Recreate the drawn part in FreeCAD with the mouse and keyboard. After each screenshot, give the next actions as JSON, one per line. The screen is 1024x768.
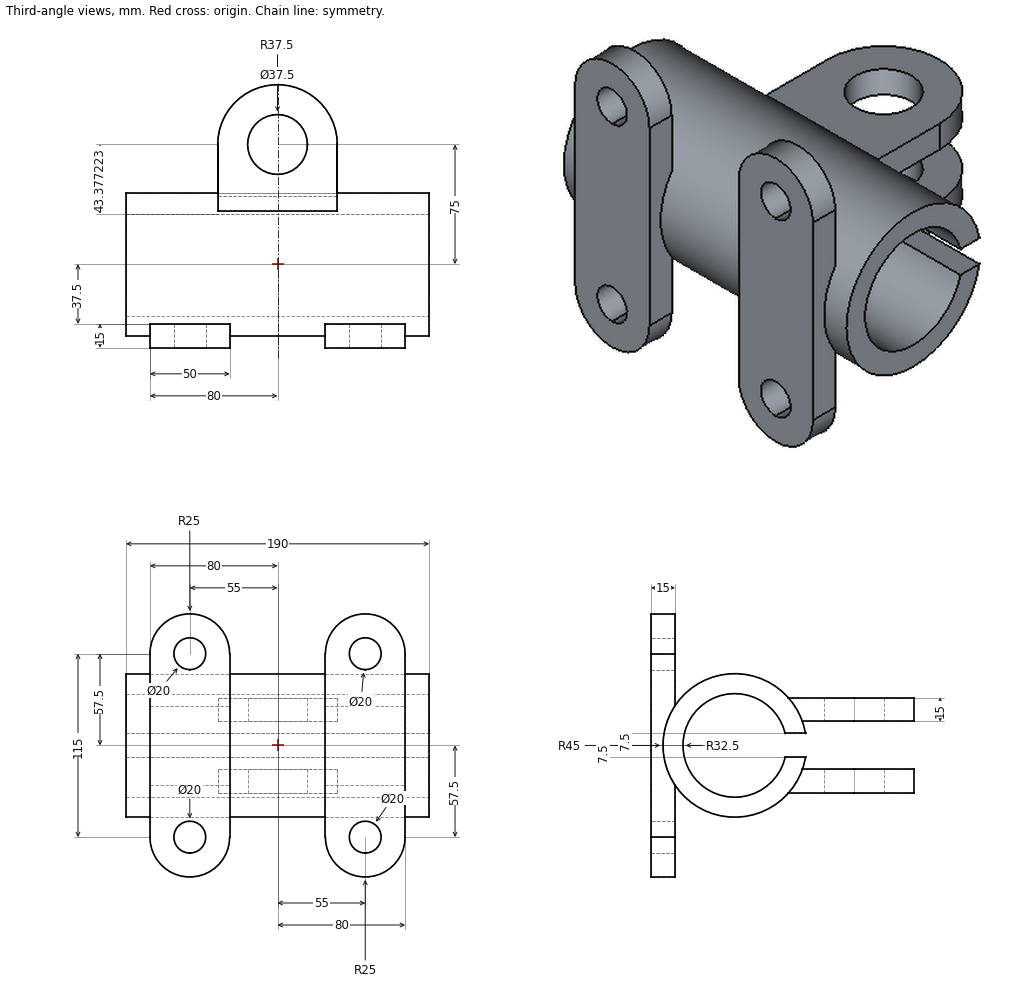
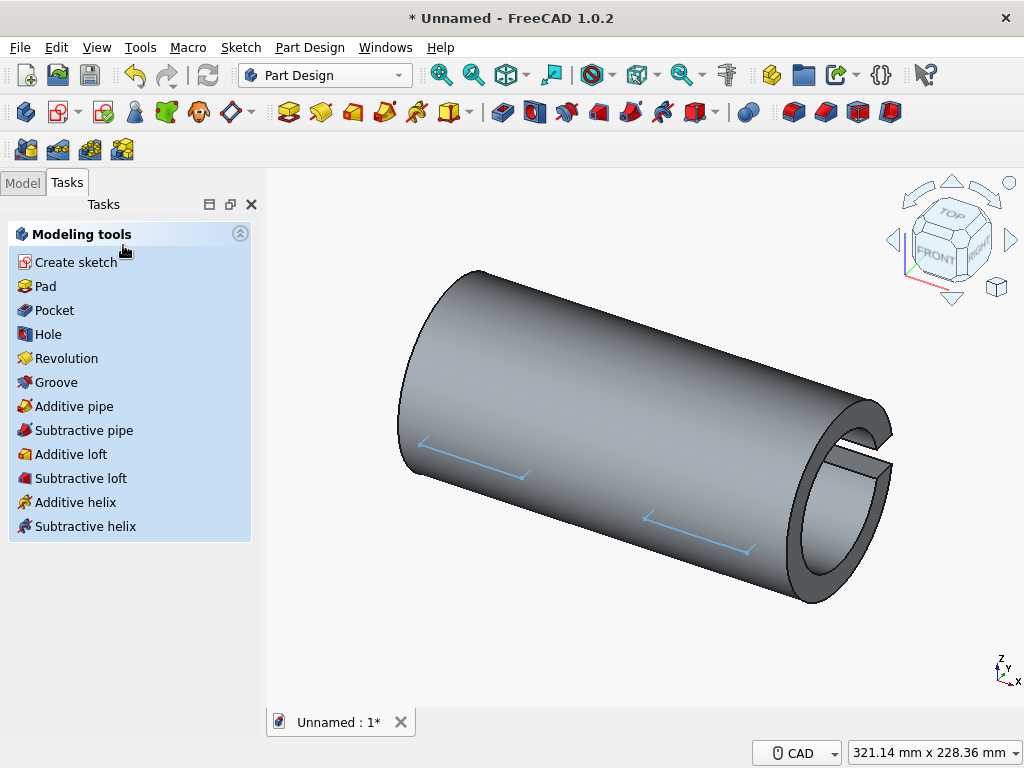
{"action": "left_click", "coordinate": [290, 112]}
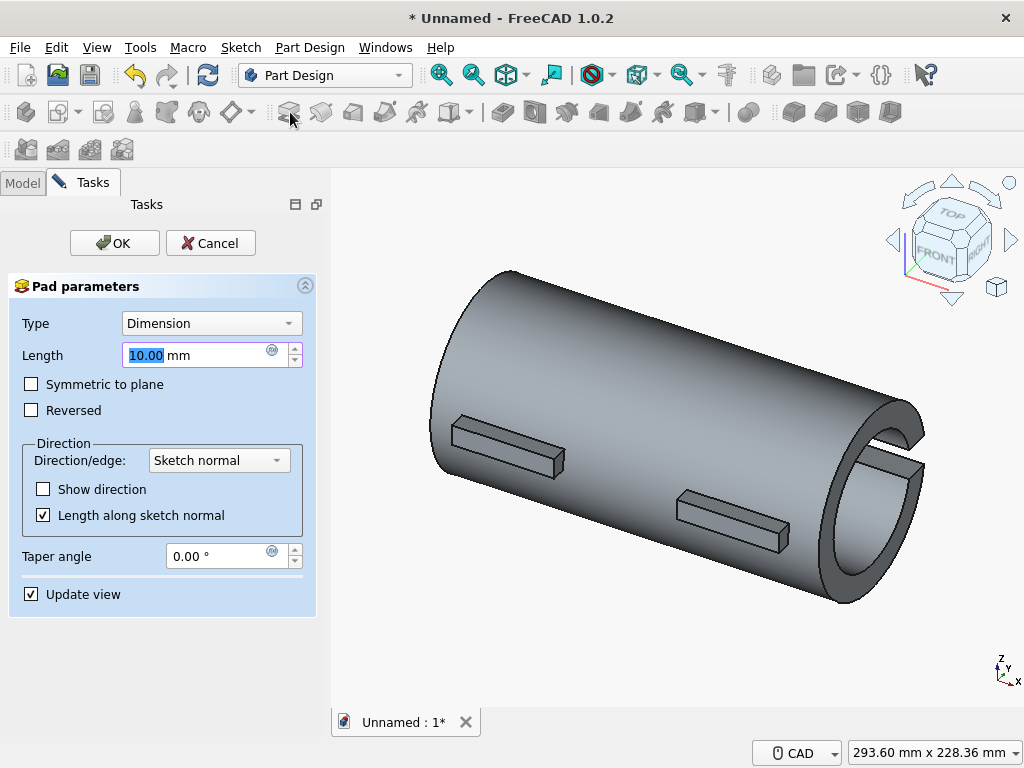
{"action": "type", "text": "115"}
{"action": "key", "text": "Tab"}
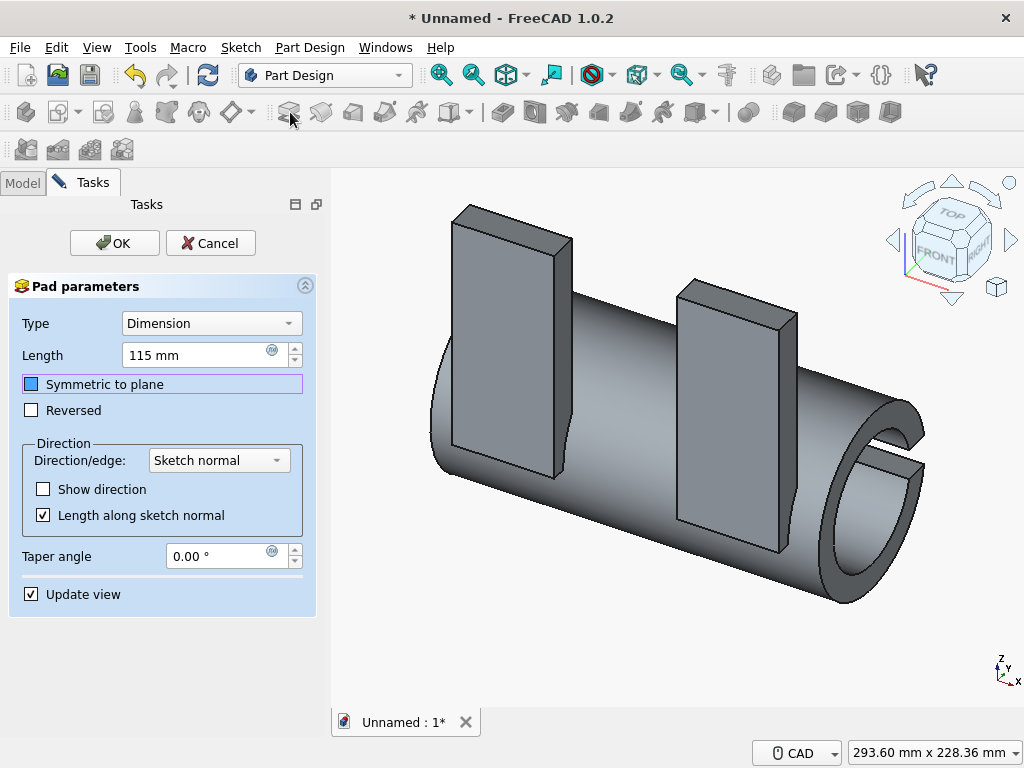
{"action": "left_click", "coordinate": [30, 384]}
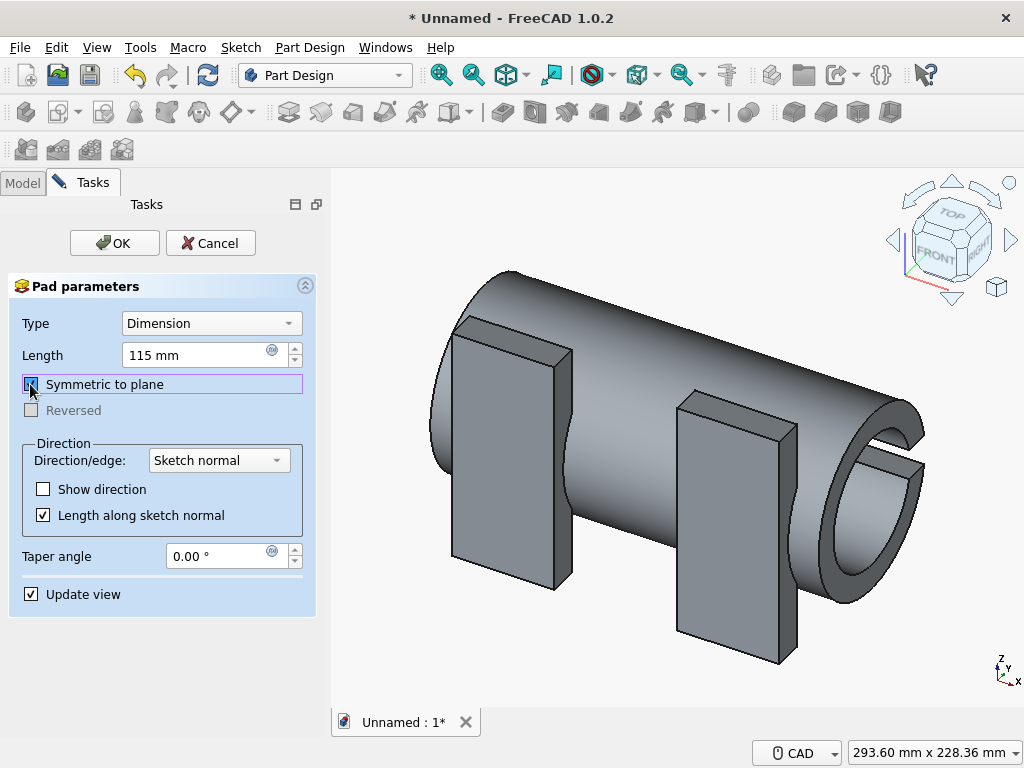
{"action": "left_click", "coordinate": [115, 243]}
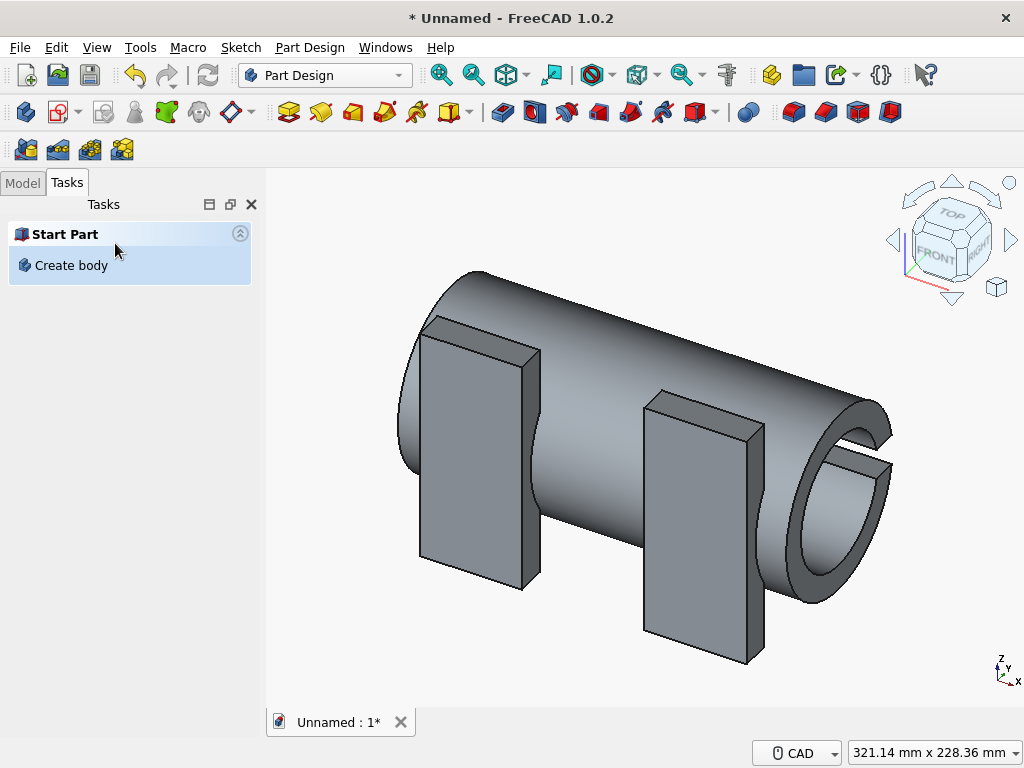
{"action": "left_click", "coordinate": [471, 429]}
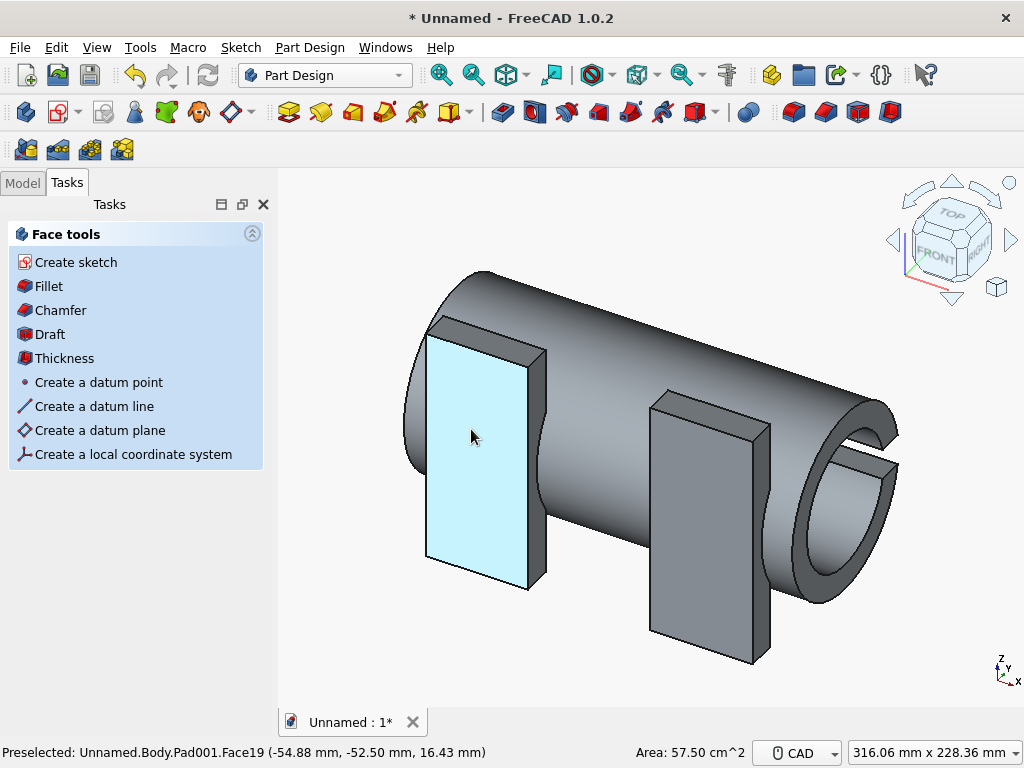
{"action": "left_click", "coordinate": [58, 112]}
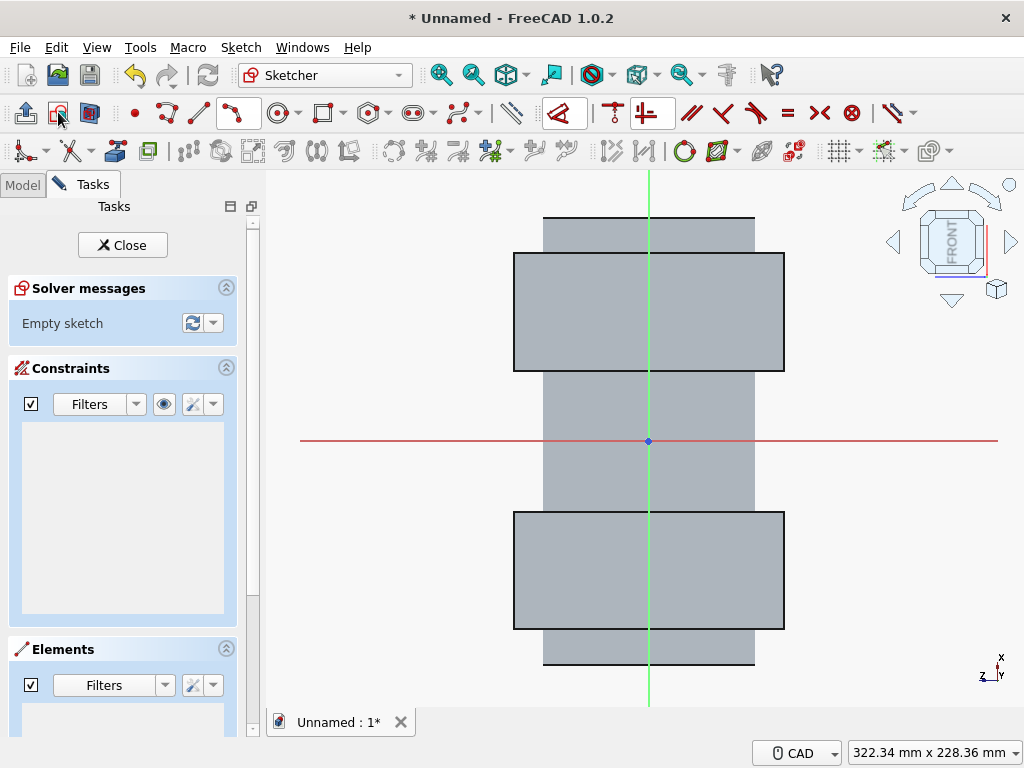
{"action": "scroll", "coordinate": [522, 653], "scroll_direction": "up", "scroll_amount": 3}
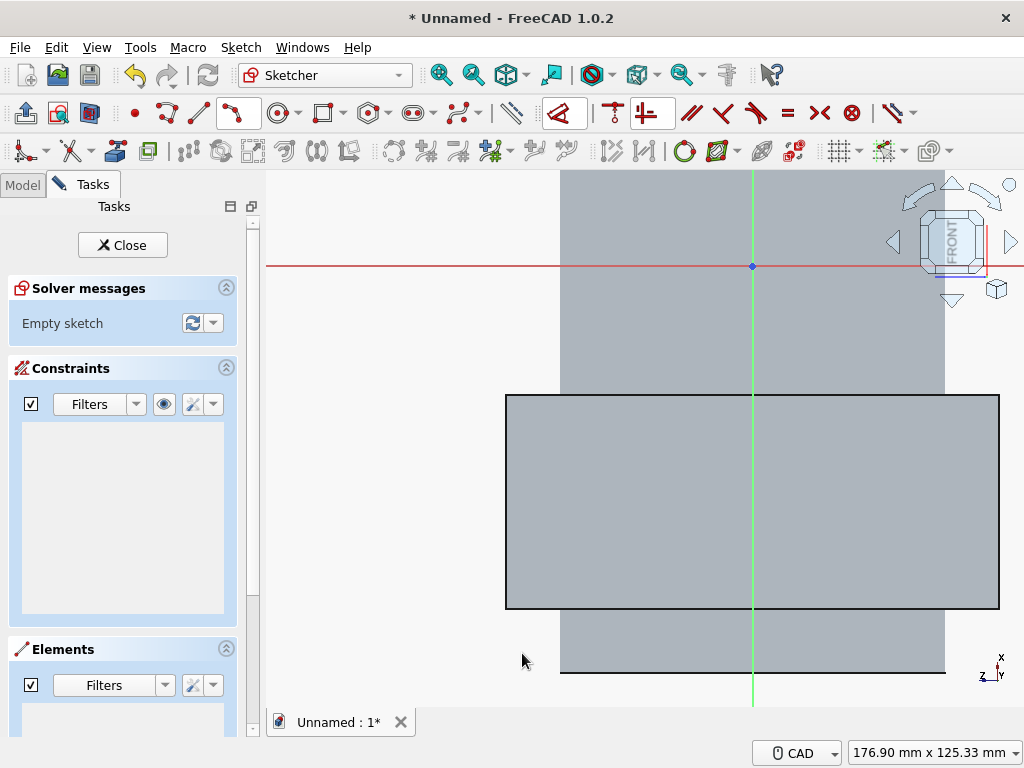
{"action": "left_click", "coordinate": [200, 114]}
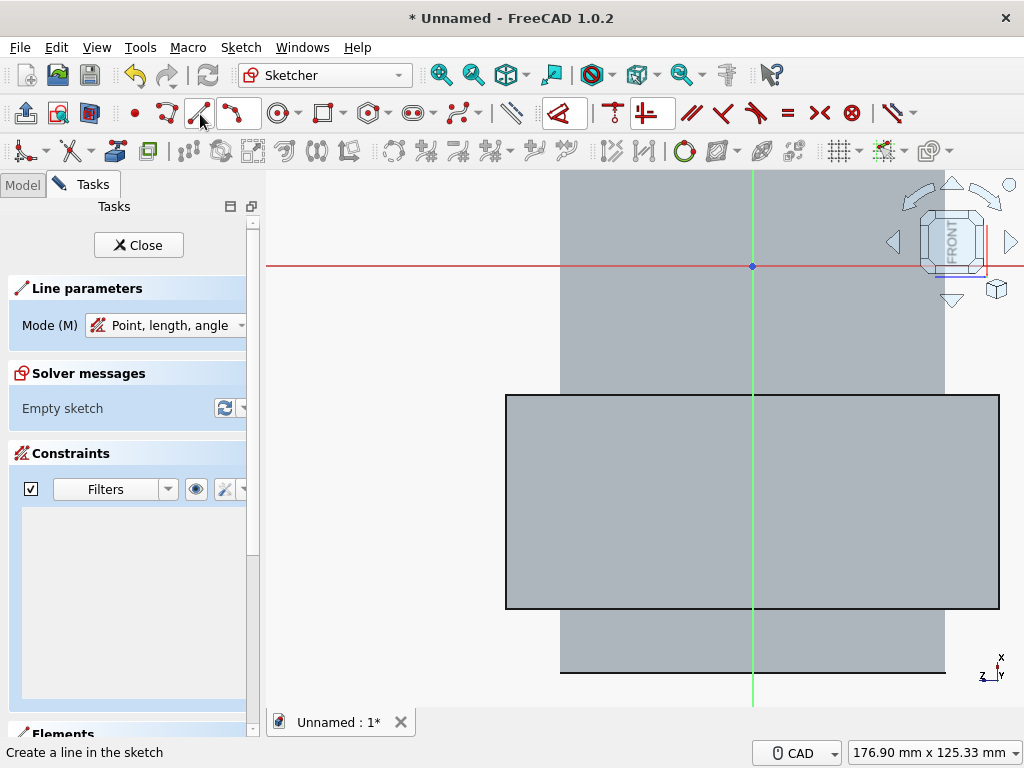
{"action": "left_click", "coordinate": [506, 609]}
{"action": "left_click", "coordinate": [506, 395]}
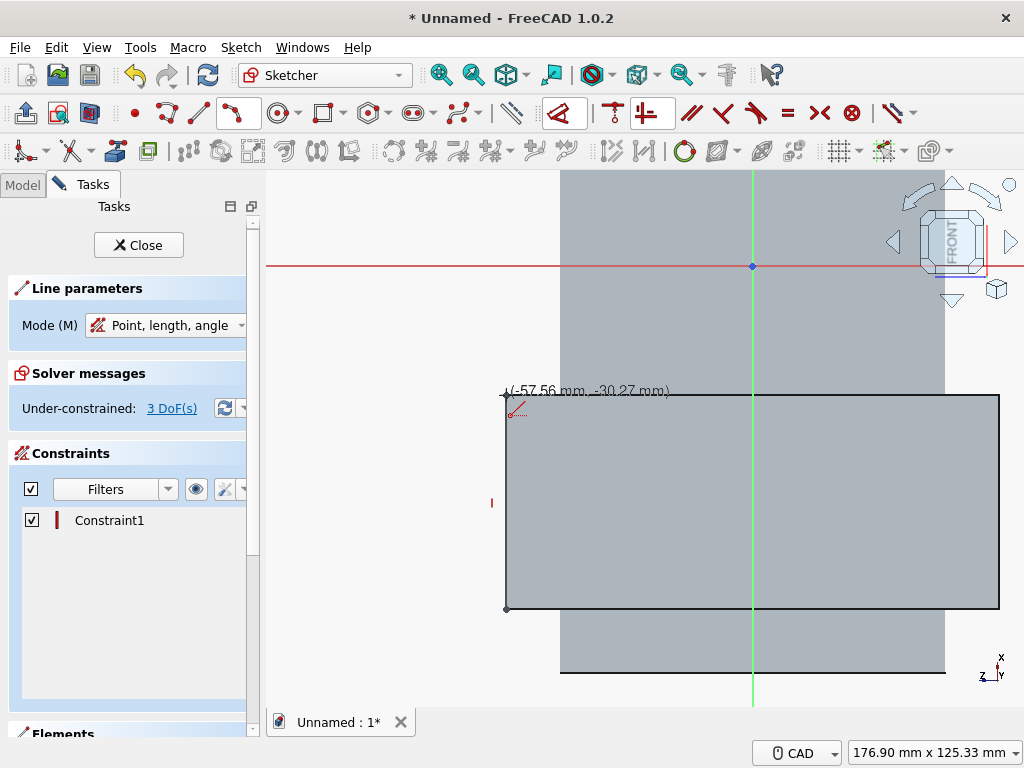
{"action": "left_click", "coordinate": [232, 114]}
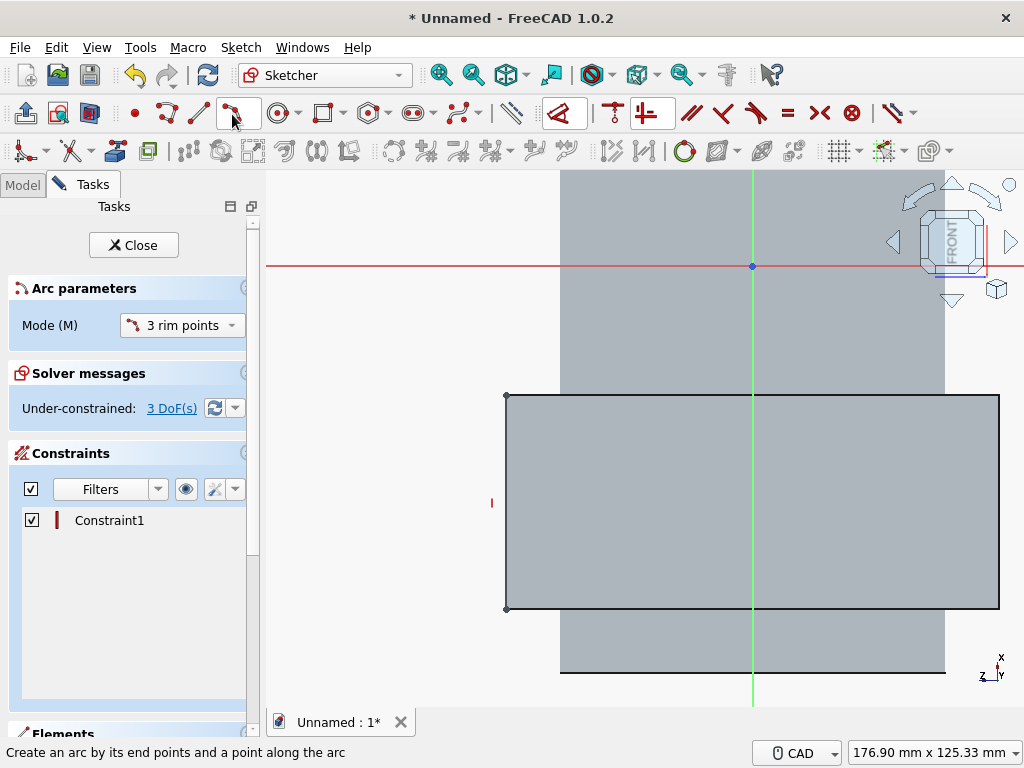
{"action": "left_click", "coordinate": [506, 396]}
{"action": "left_click", "coordinate": [506, 610]}
{"action": "left_click", "coordinate": [399, 502]}
{"action": "key", "text": "Escape"}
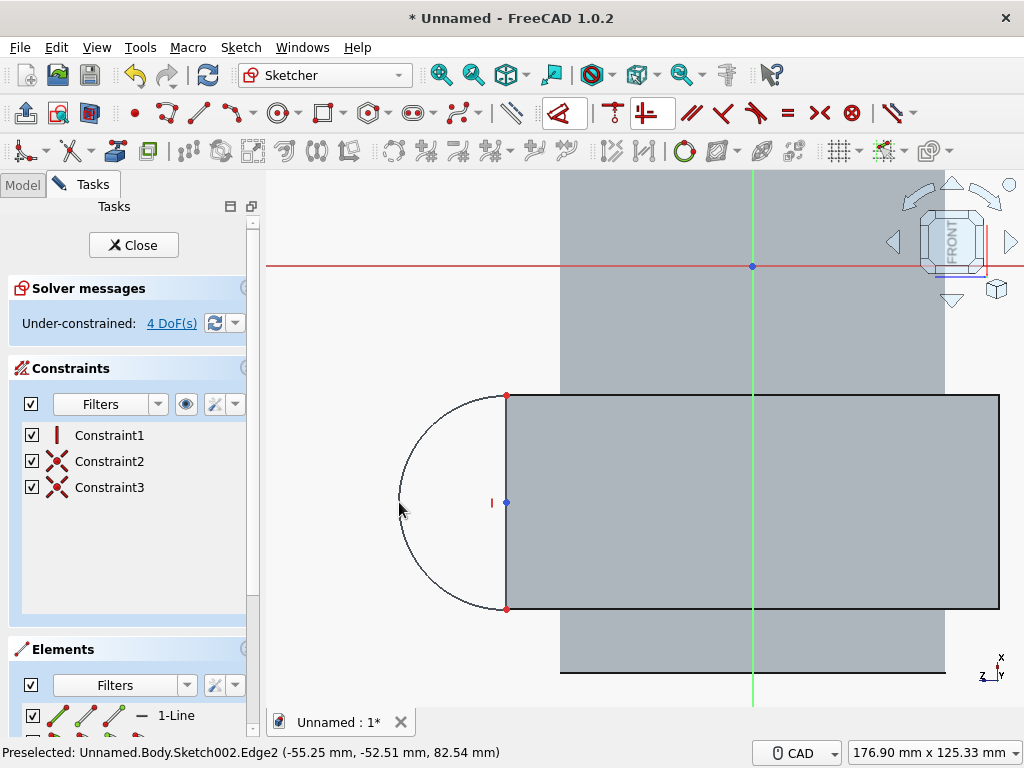
{"action": "left_click", "coordinate": [419, 440]}